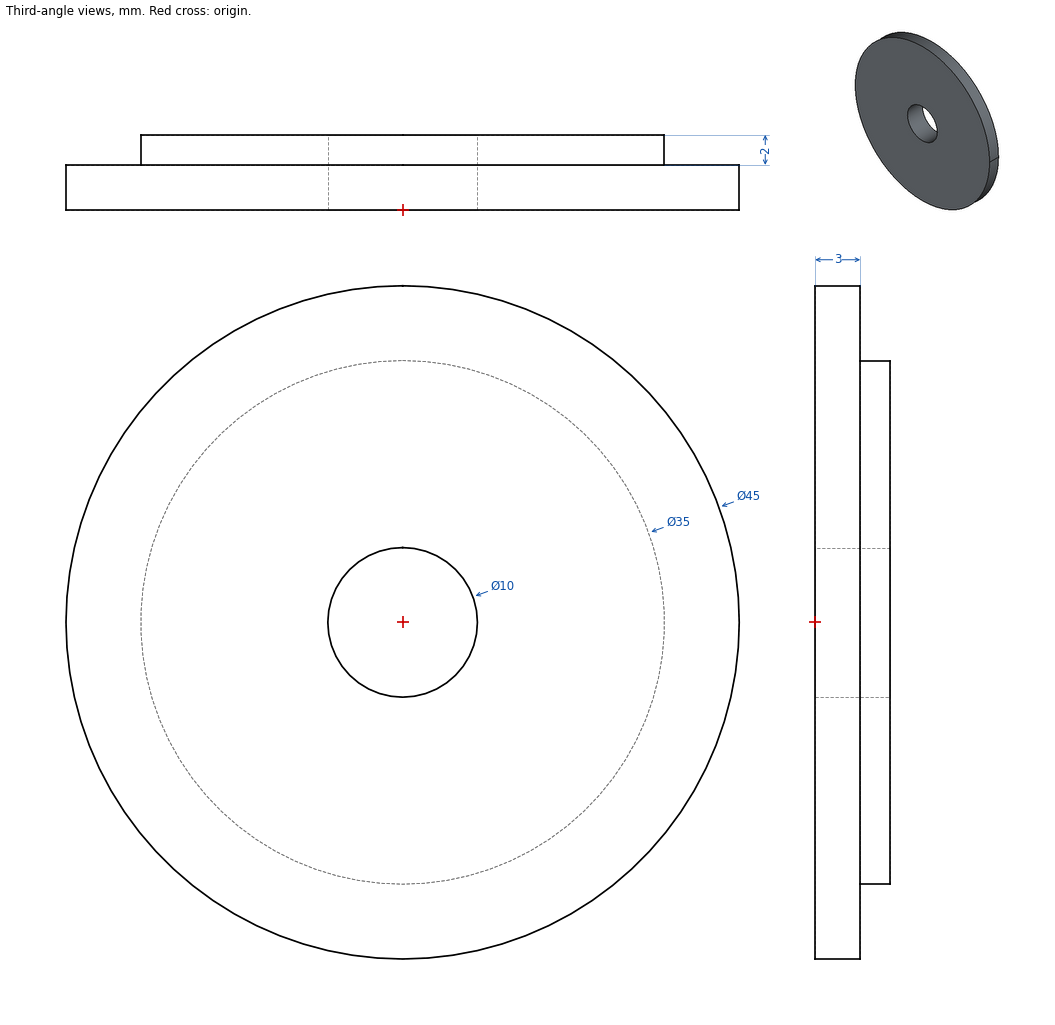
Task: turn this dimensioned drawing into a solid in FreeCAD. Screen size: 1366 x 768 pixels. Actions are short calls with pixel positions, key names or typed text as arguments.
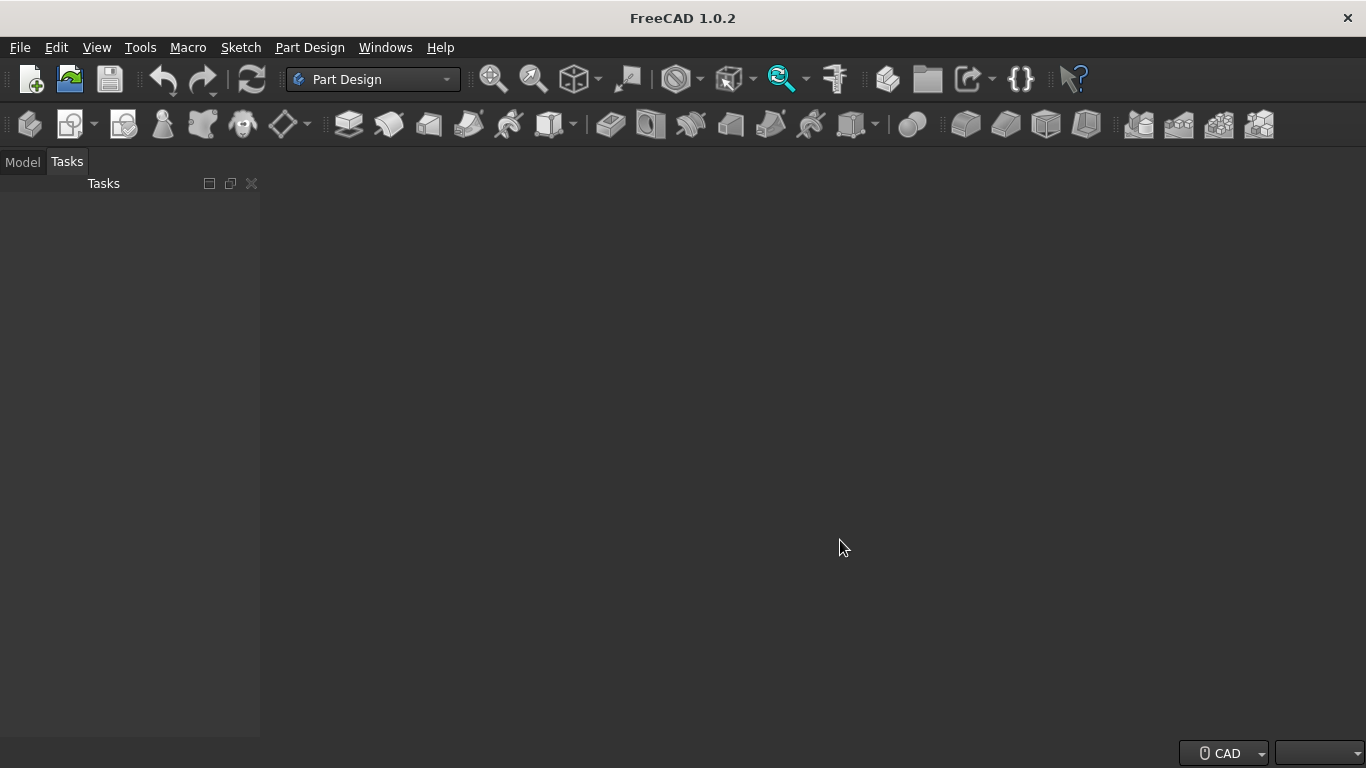
key(ctrl+n)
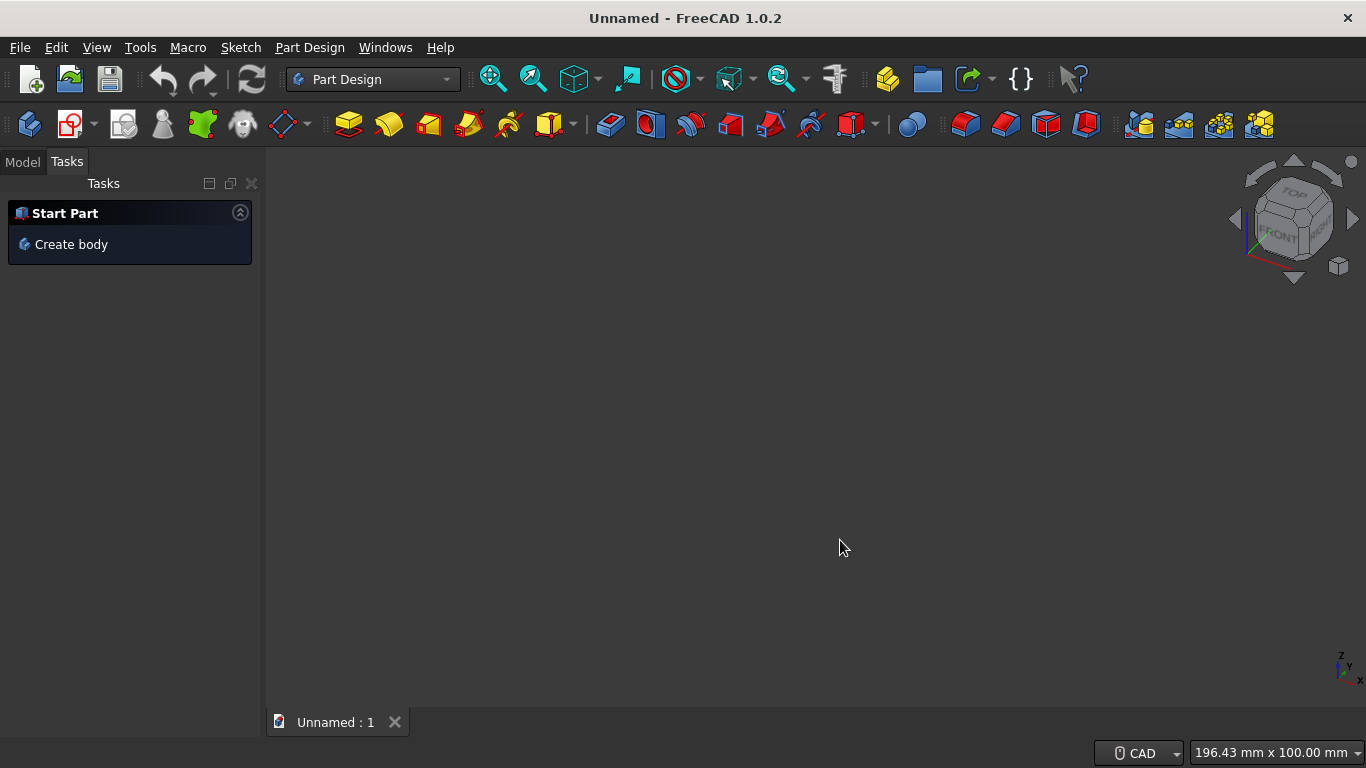
click(70, 124)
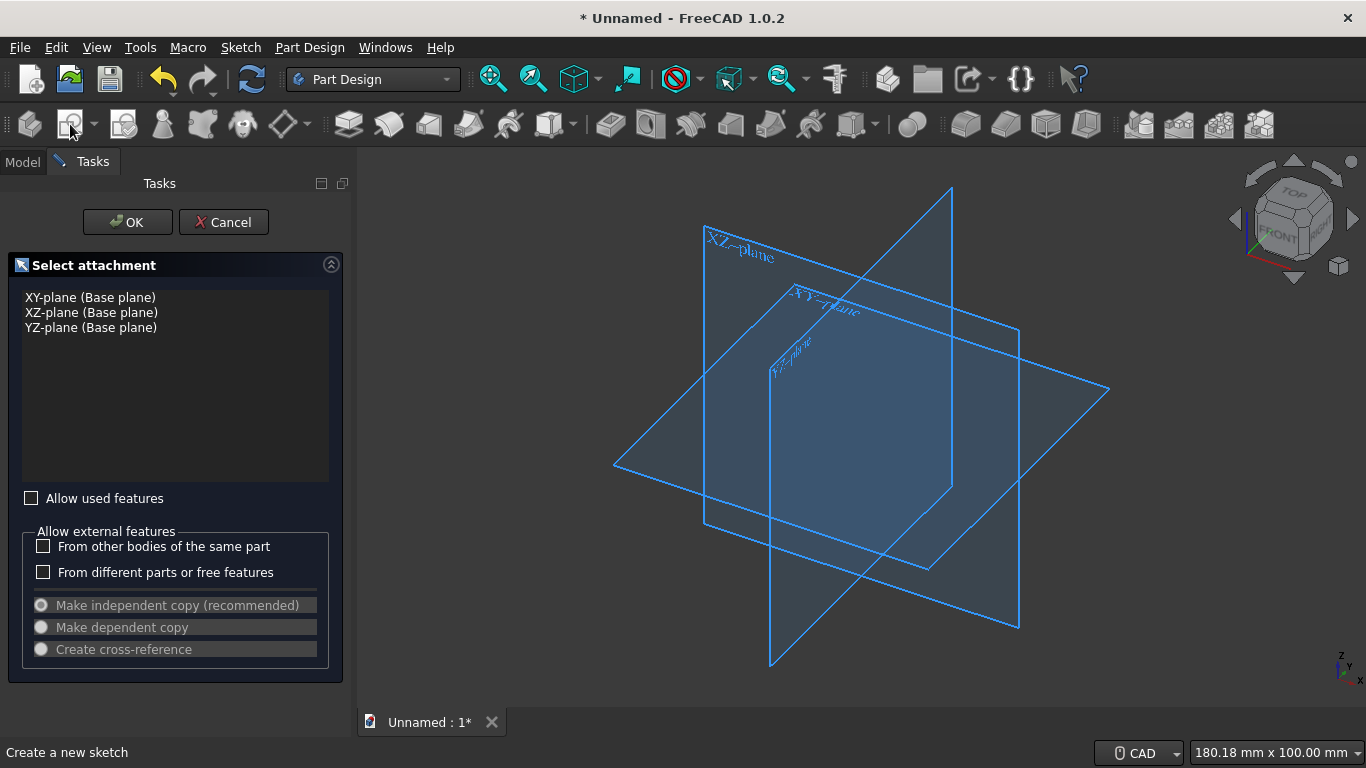
click(82, 312)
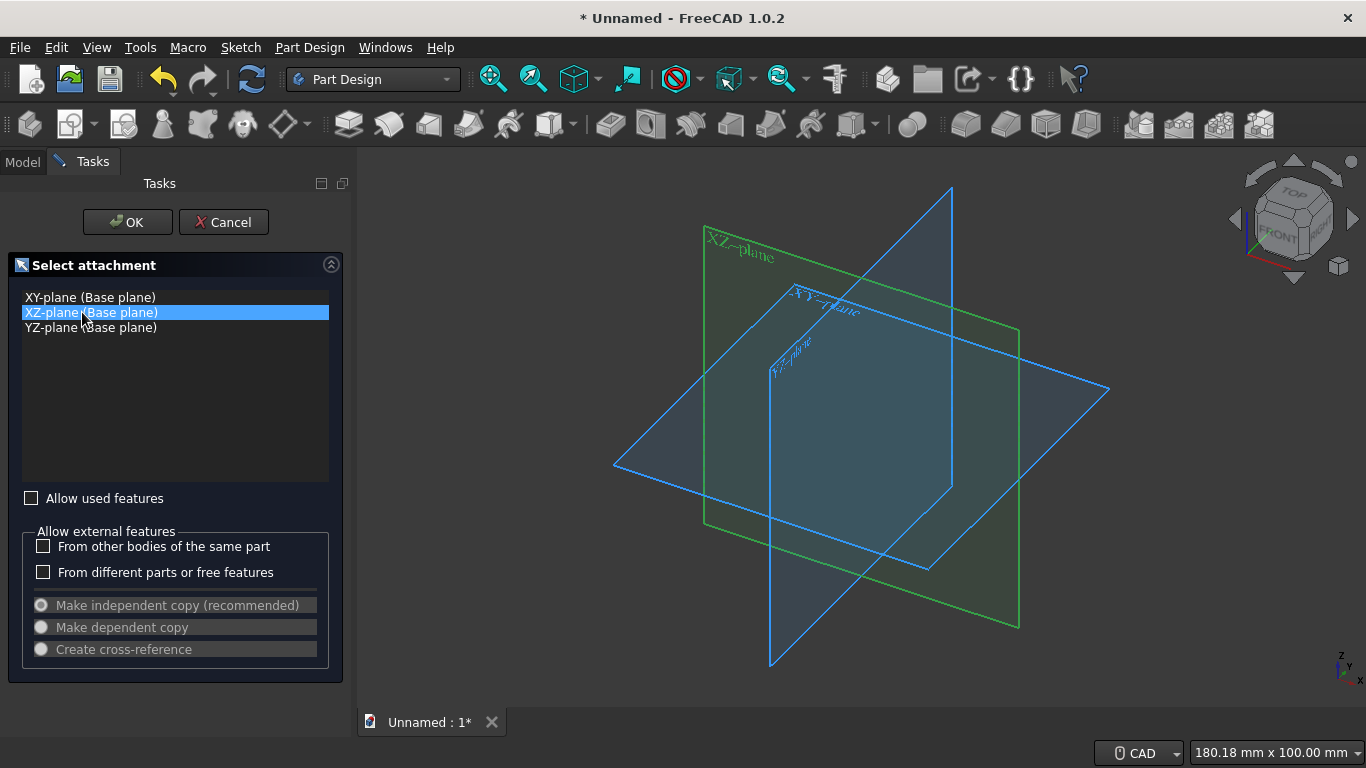
click(128, 222)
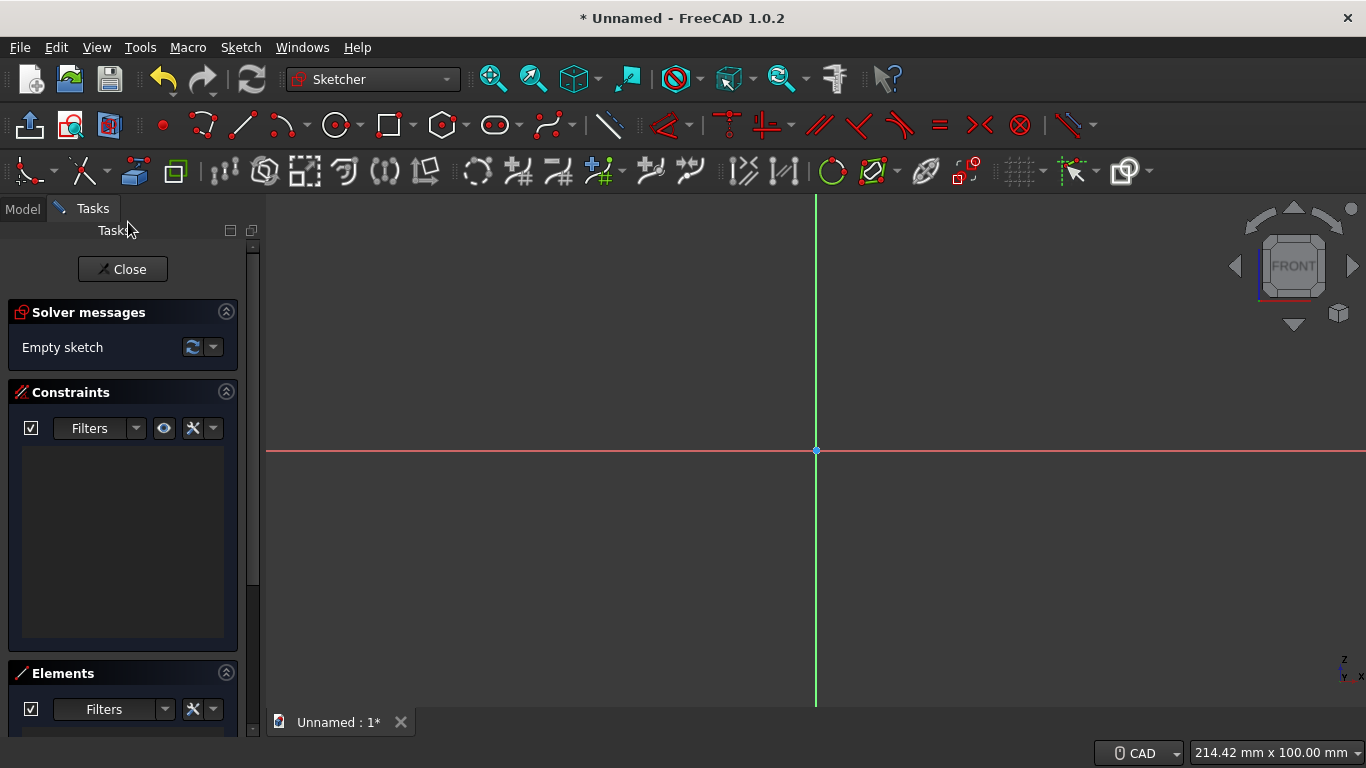
scroll(955, 451, up, 2)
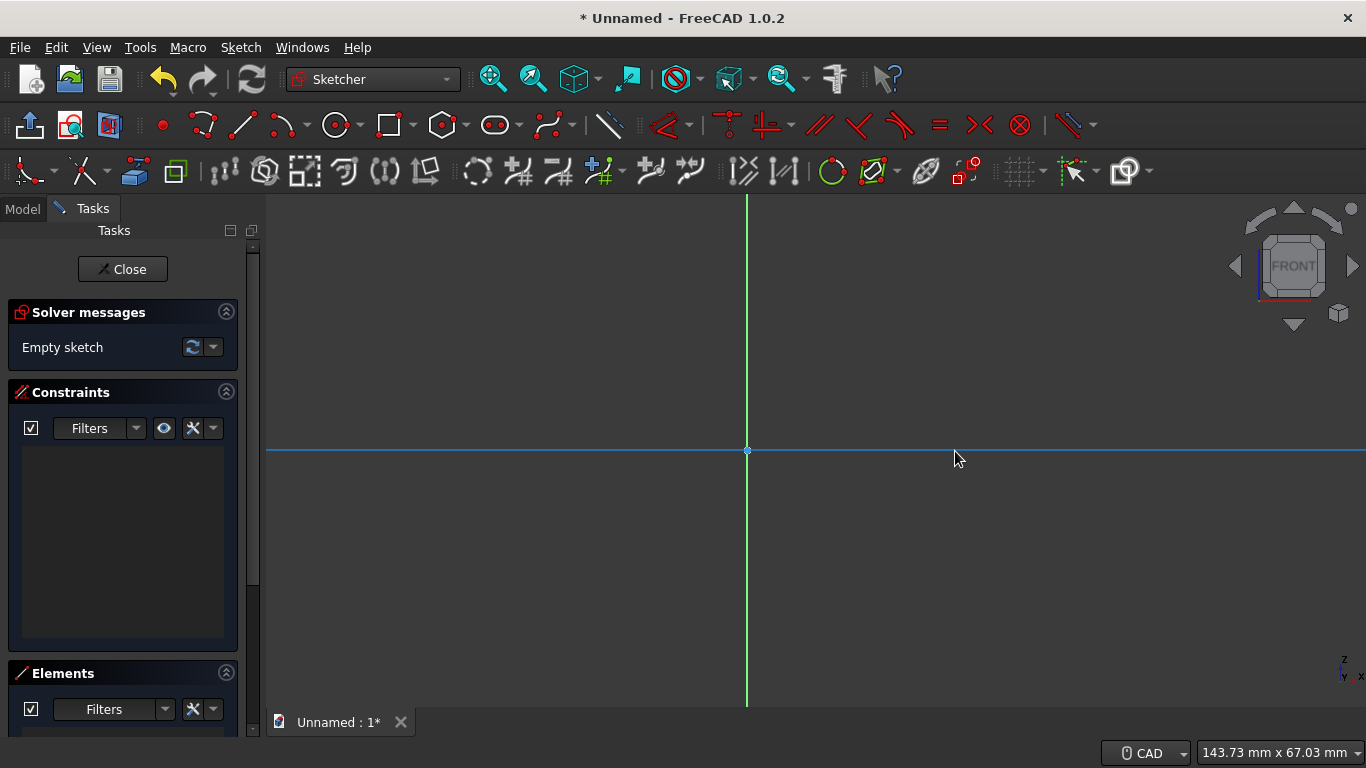
key(g)
key(c)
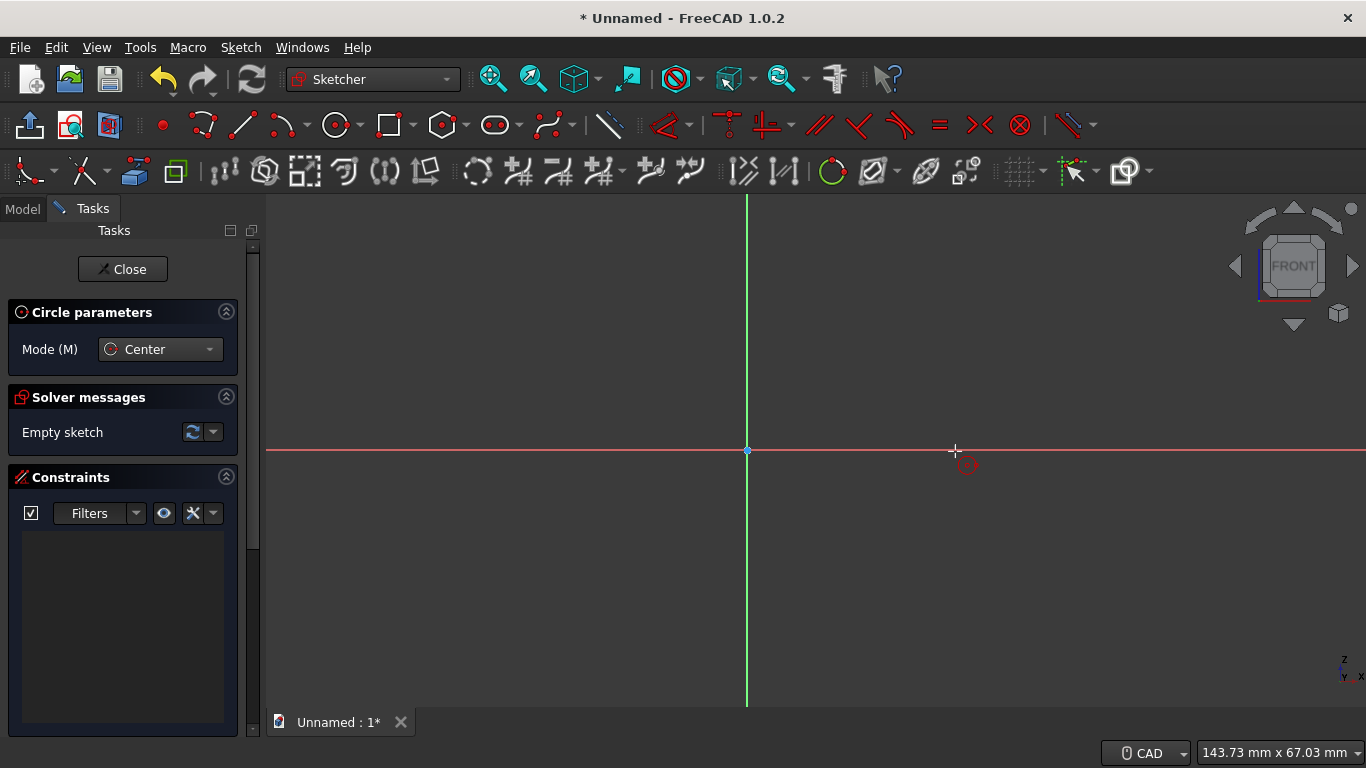
click(747, 450)
click(869, 328)
key(Escape)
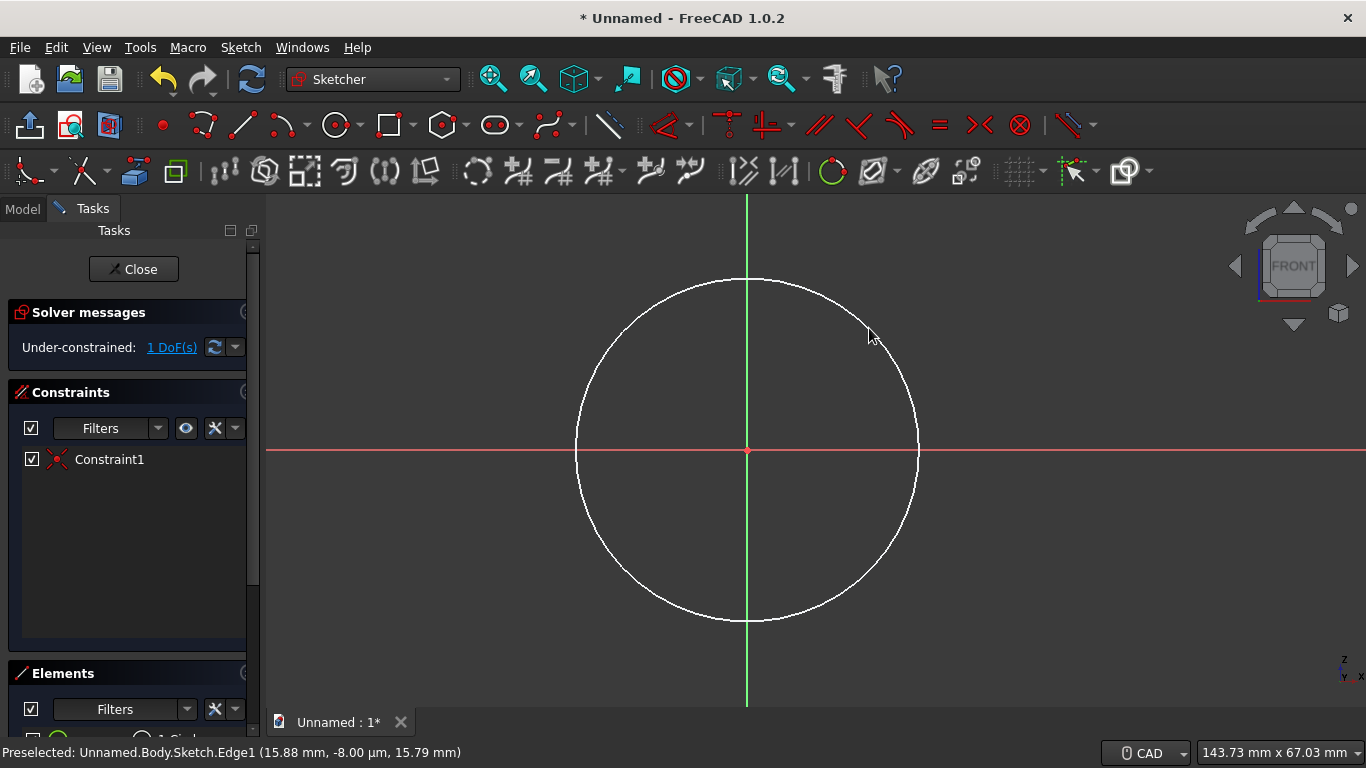
key(d)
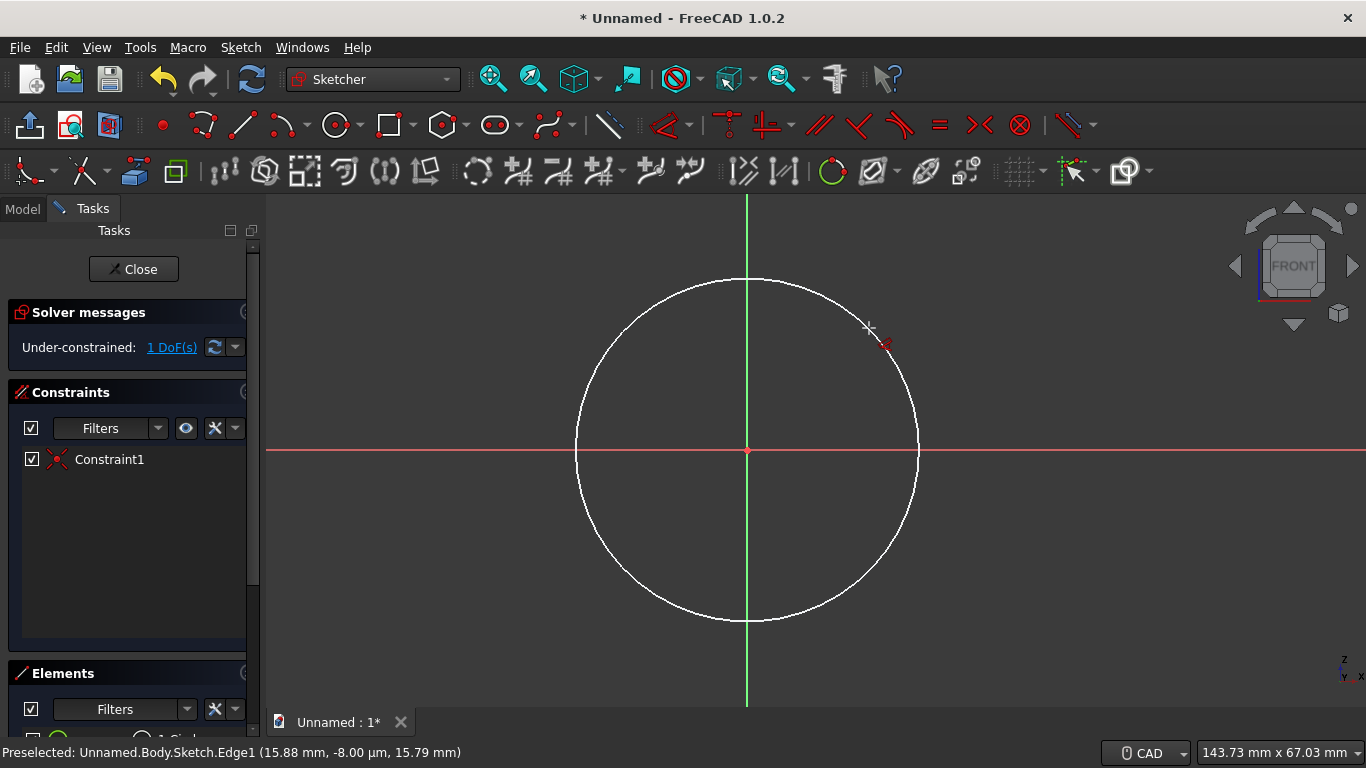
click(868, 328)
click(891, 305)